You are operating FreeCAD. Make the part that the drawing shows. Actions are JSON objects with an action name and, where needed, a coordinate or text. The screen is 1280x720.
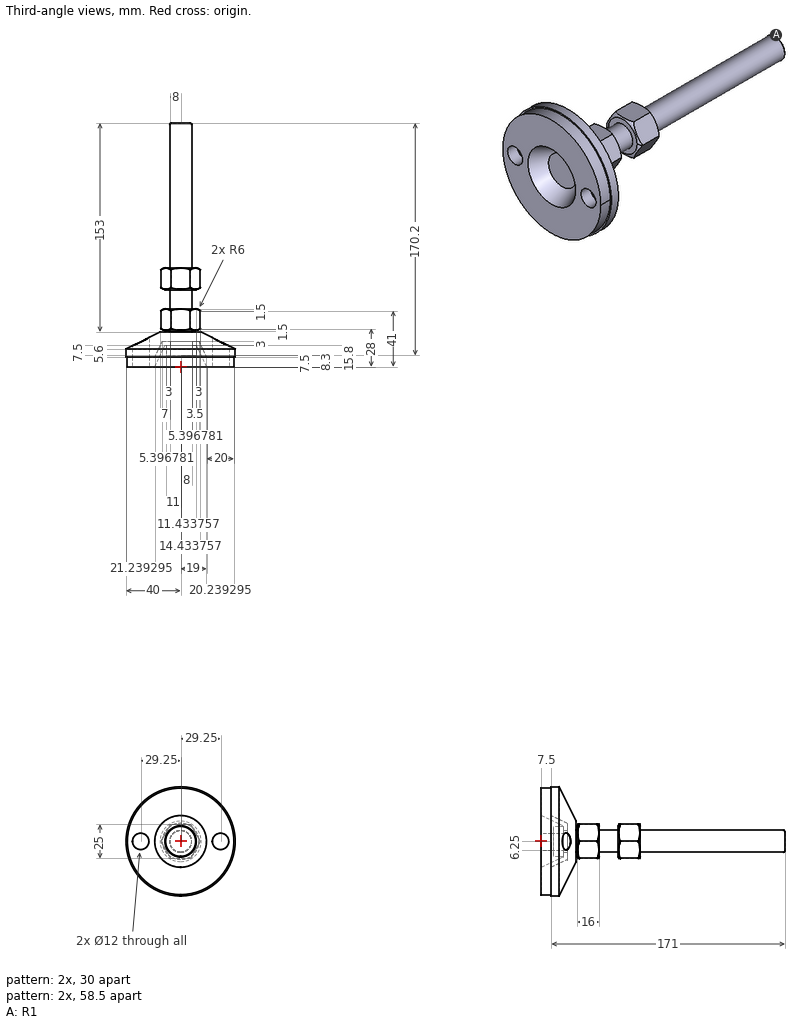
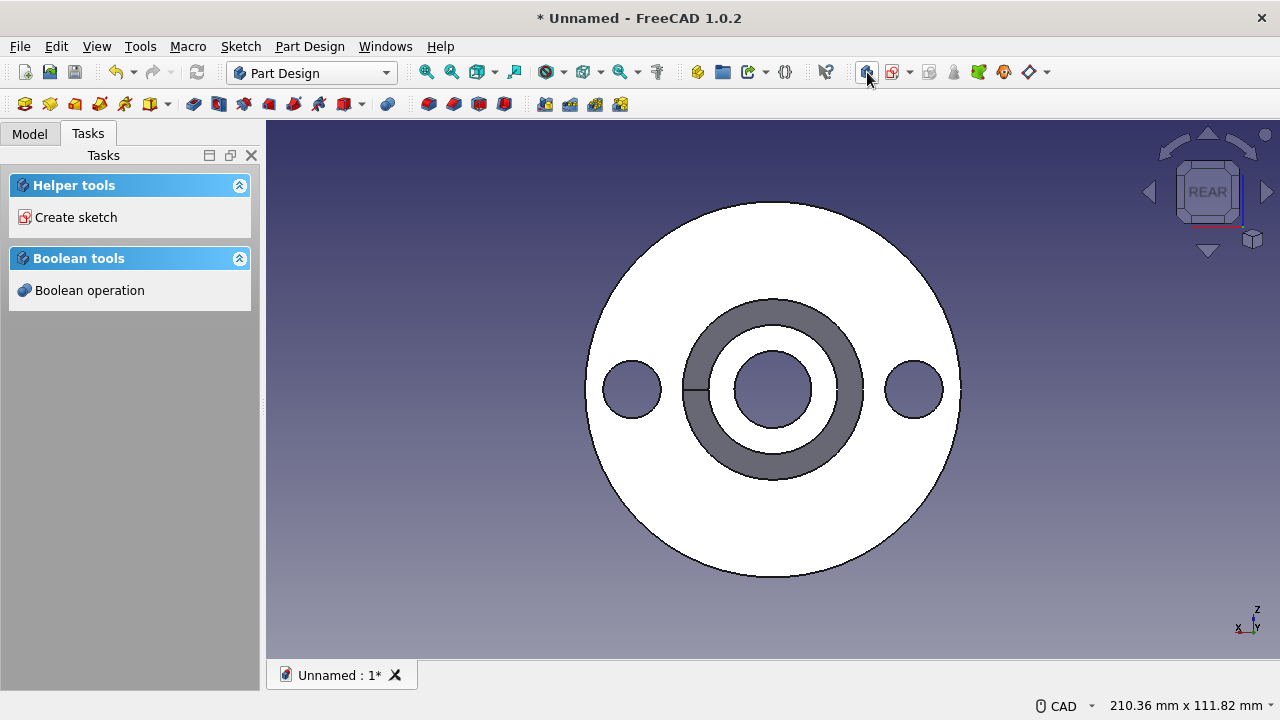
{"action": "left_click", "coordinate": [306, 619]}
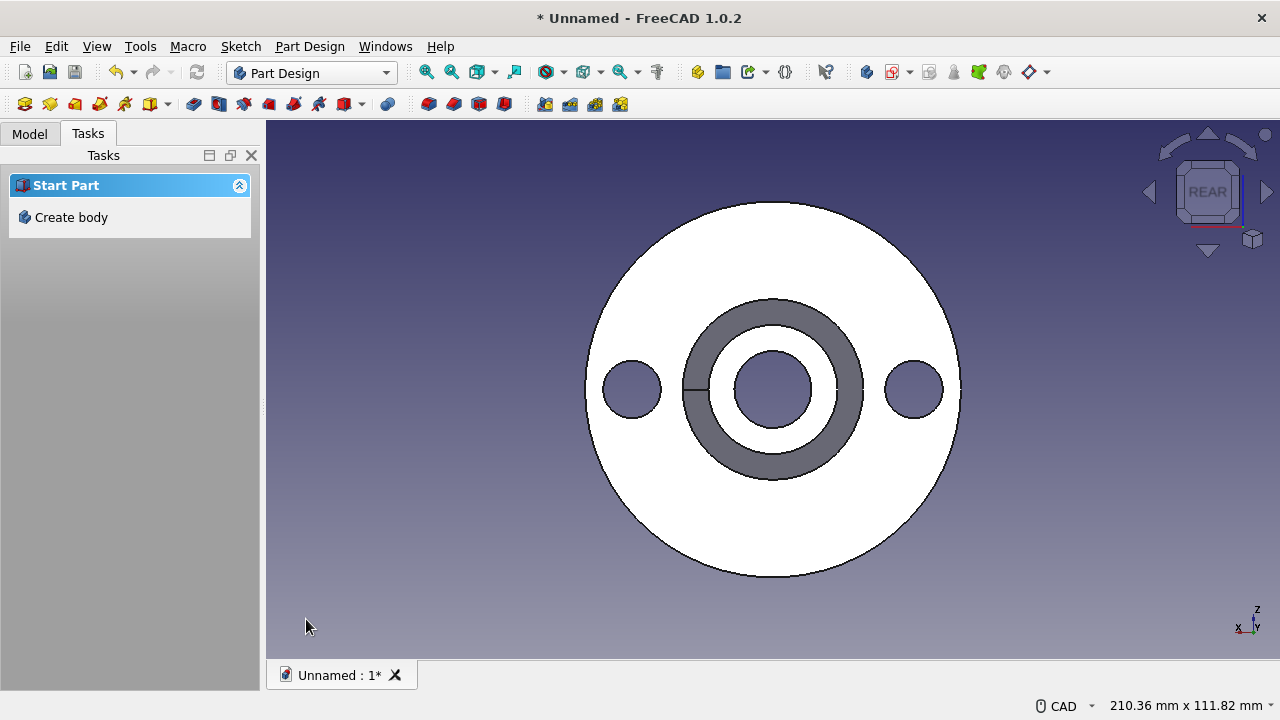
{"action": "left_click", "coordinate": [892, 72]}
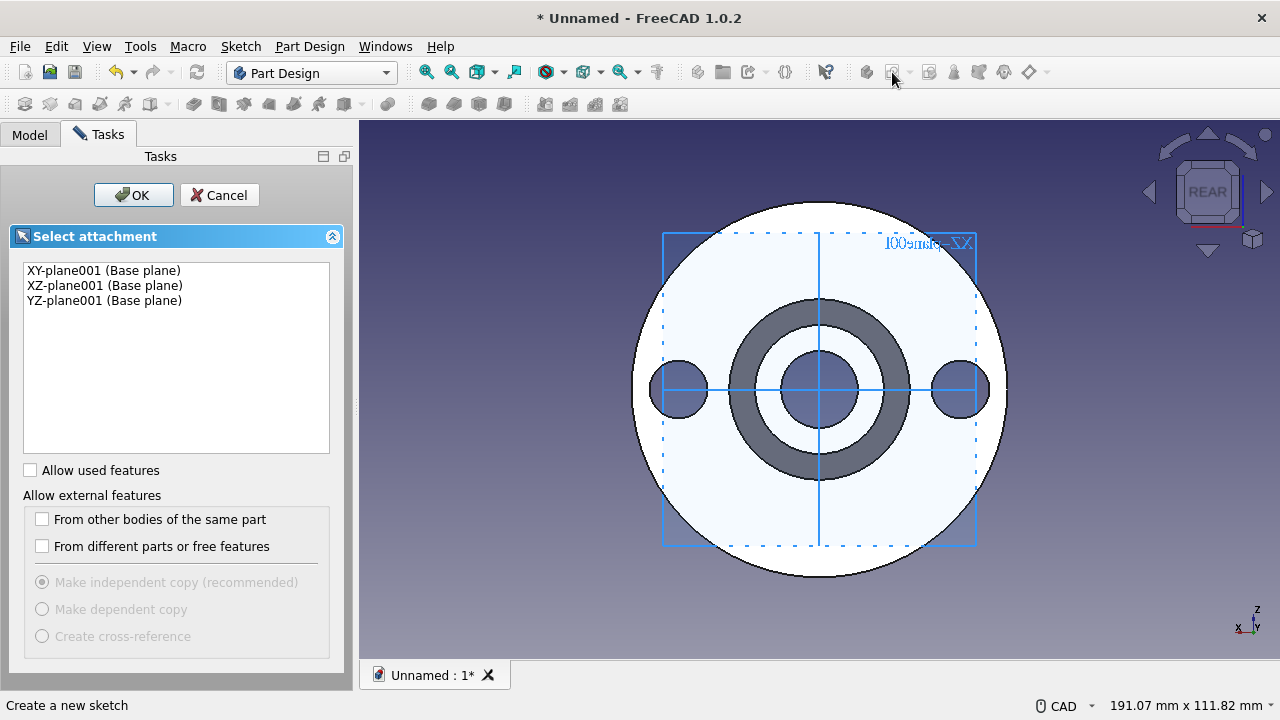
{"action": "left_click", "coordinate": [84, 270]}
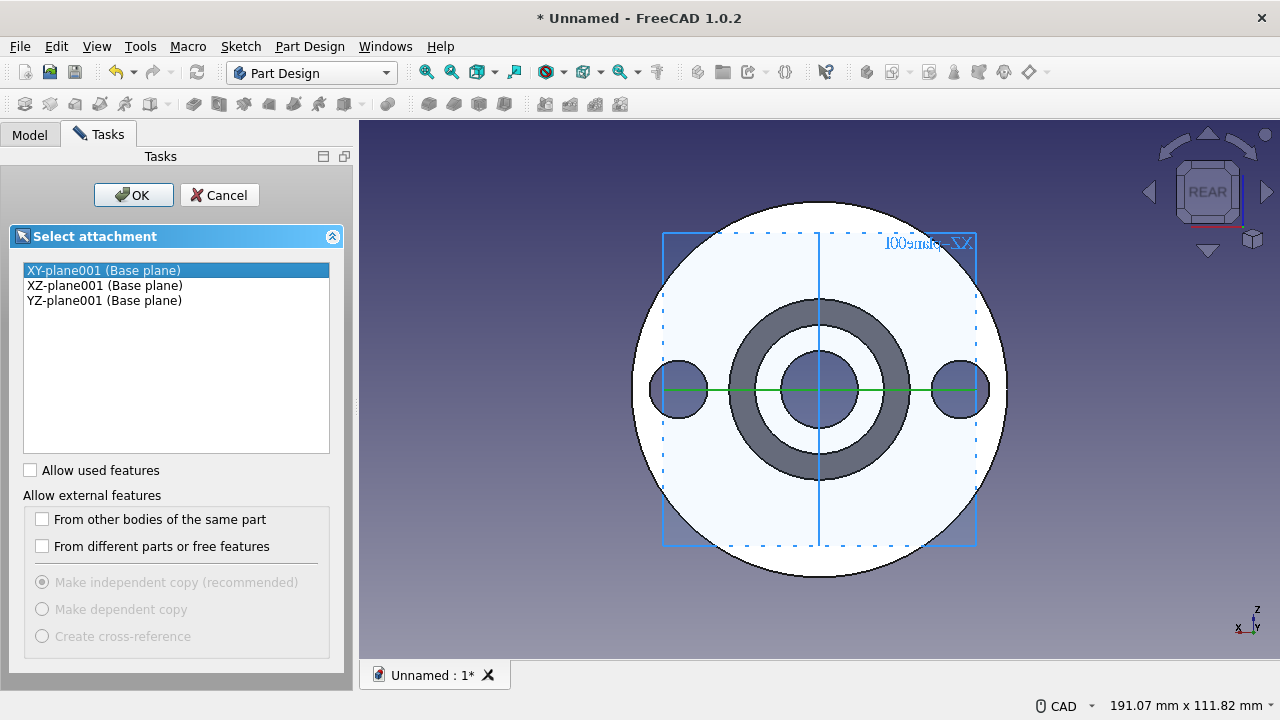
{"action": "left_click", "coordinate": [134, 195]}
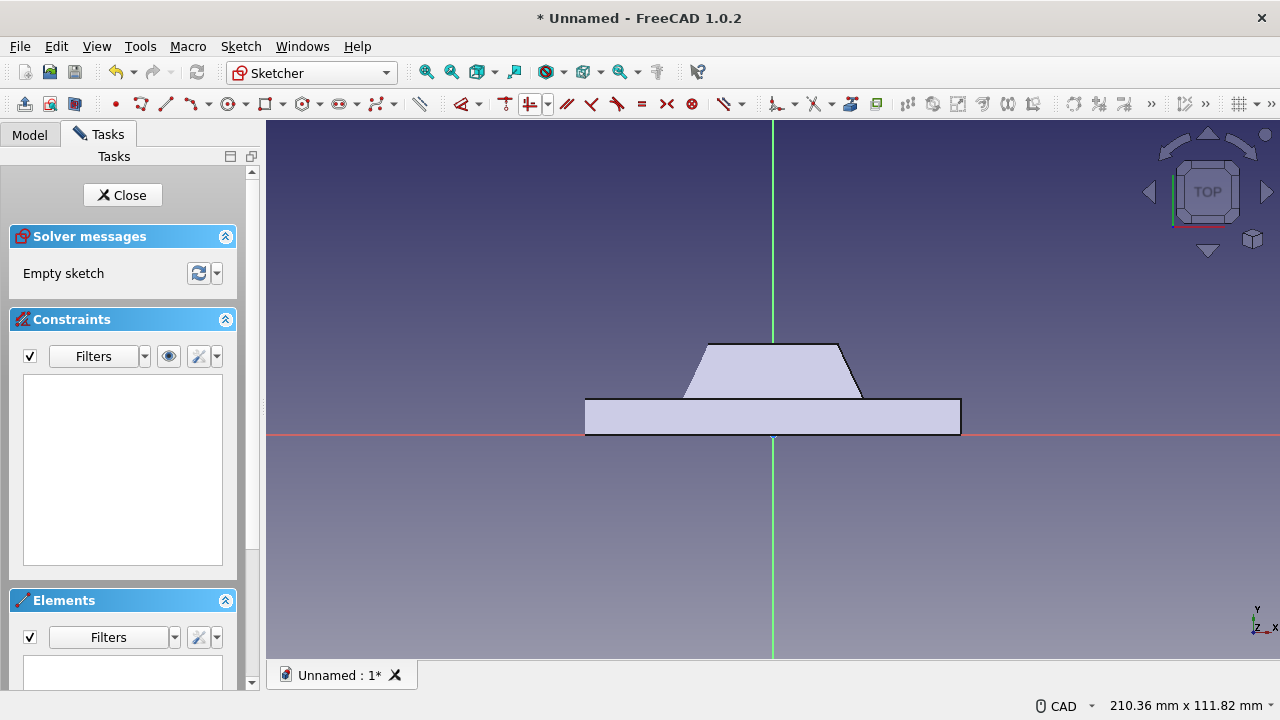
{"action": "scroll", "coordinate": [721, 614], "scroll_direction": "down", "scroll_amount": 5}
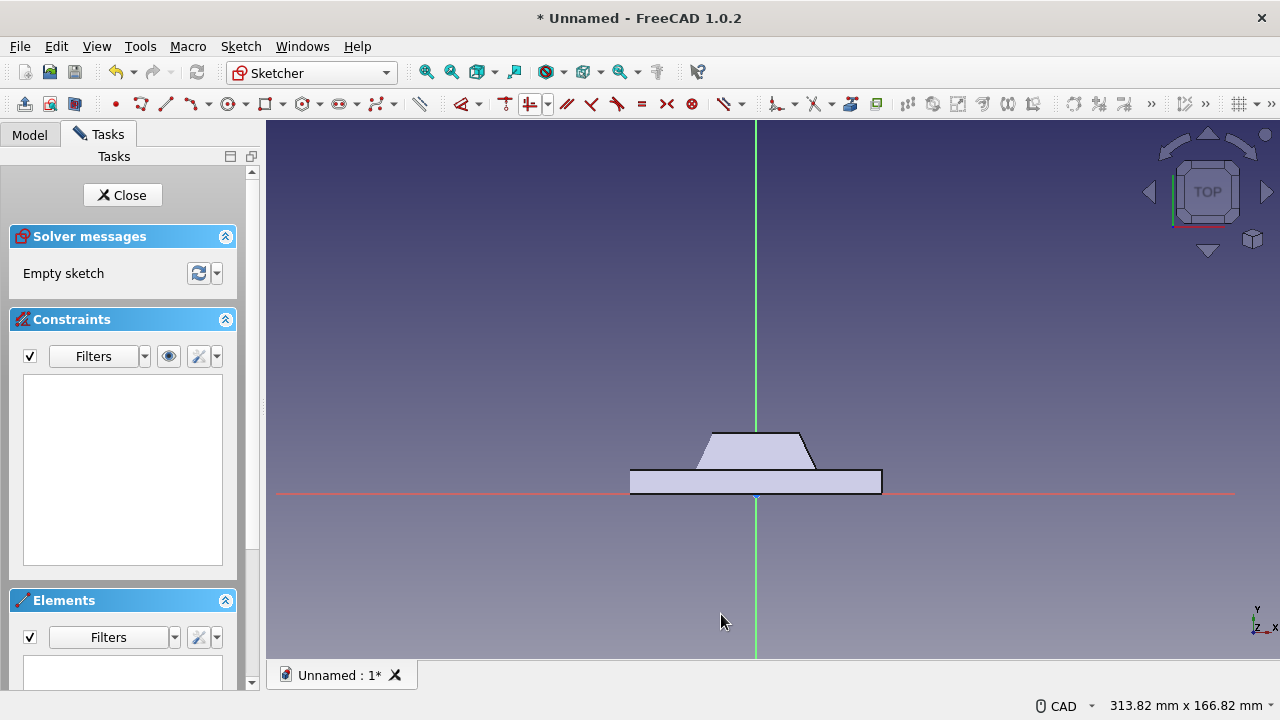
{"action": "left_click", "coordinate": [141, 104]}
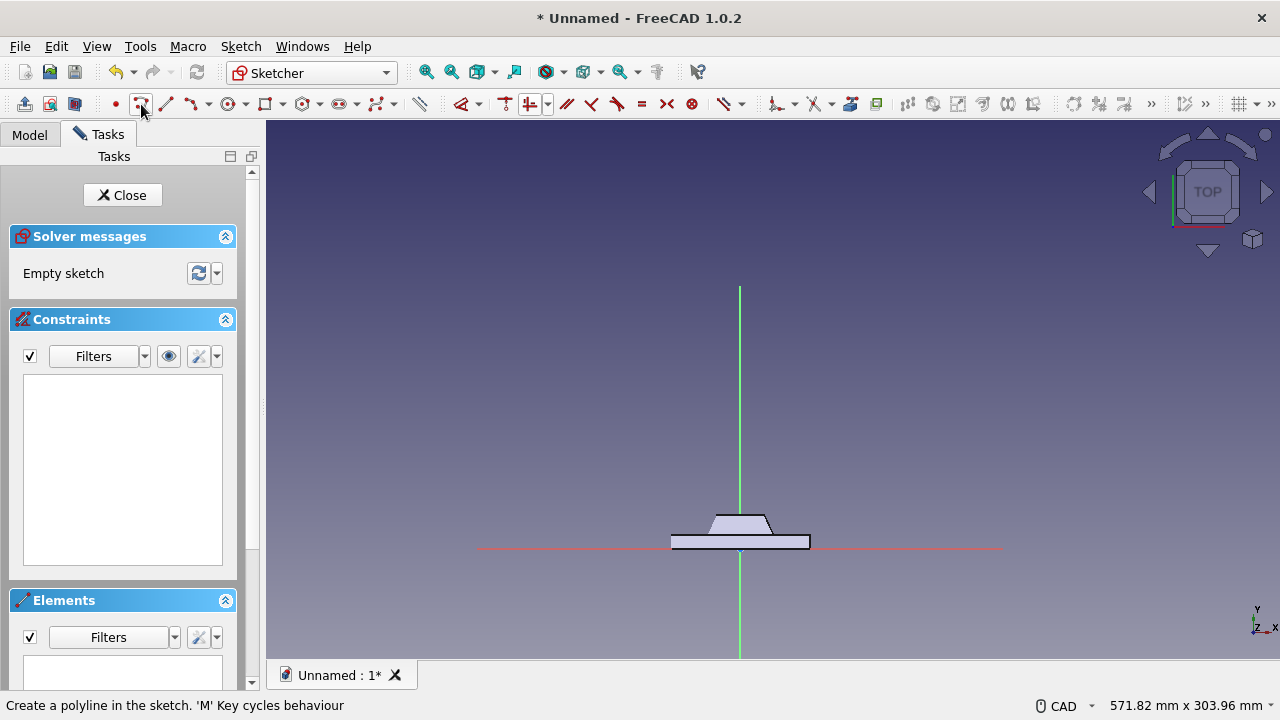
{"action": "left_click", "coordinate": [740, 534]}
{"action": "left_click", "coordinate": [731, 232]}
{"action": "left_click", "coordinate": [726, 232]}
{"action": "left_click", "coordinate": [726, 503]}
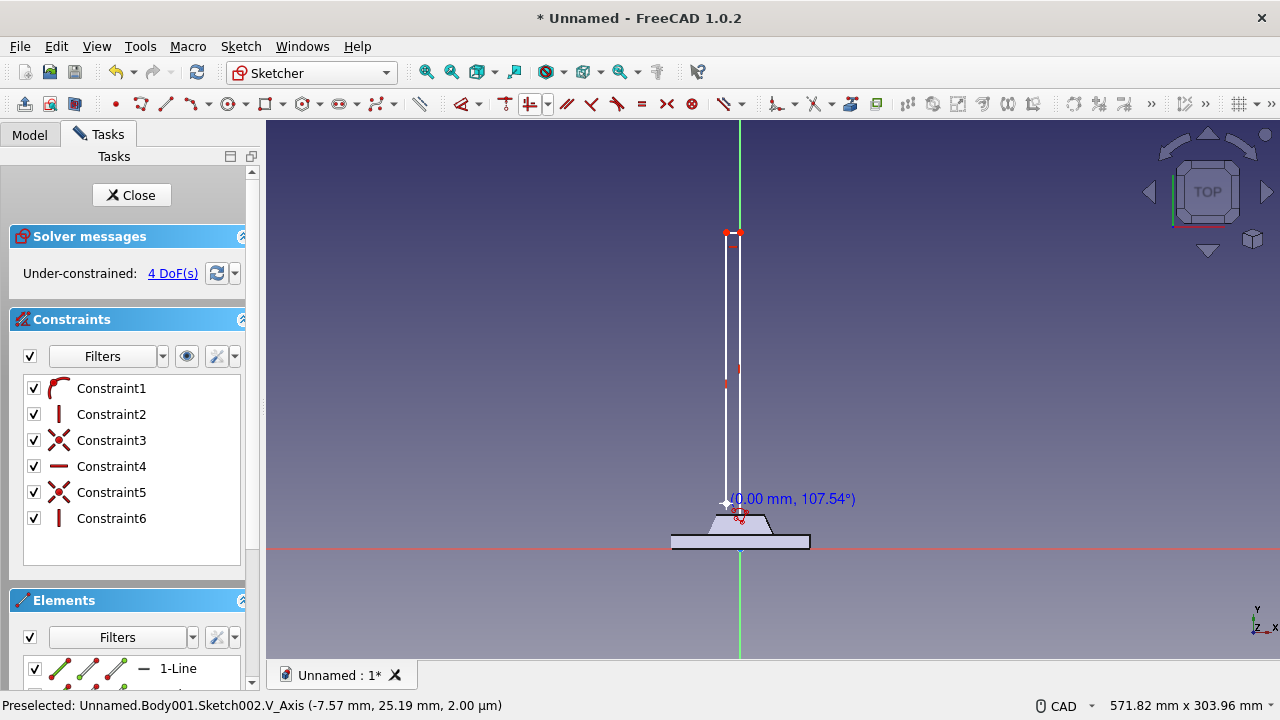
{"action": "scroll", "coordinate": [714, 503], "scroll_direction": "up", "scroll_amount": 2}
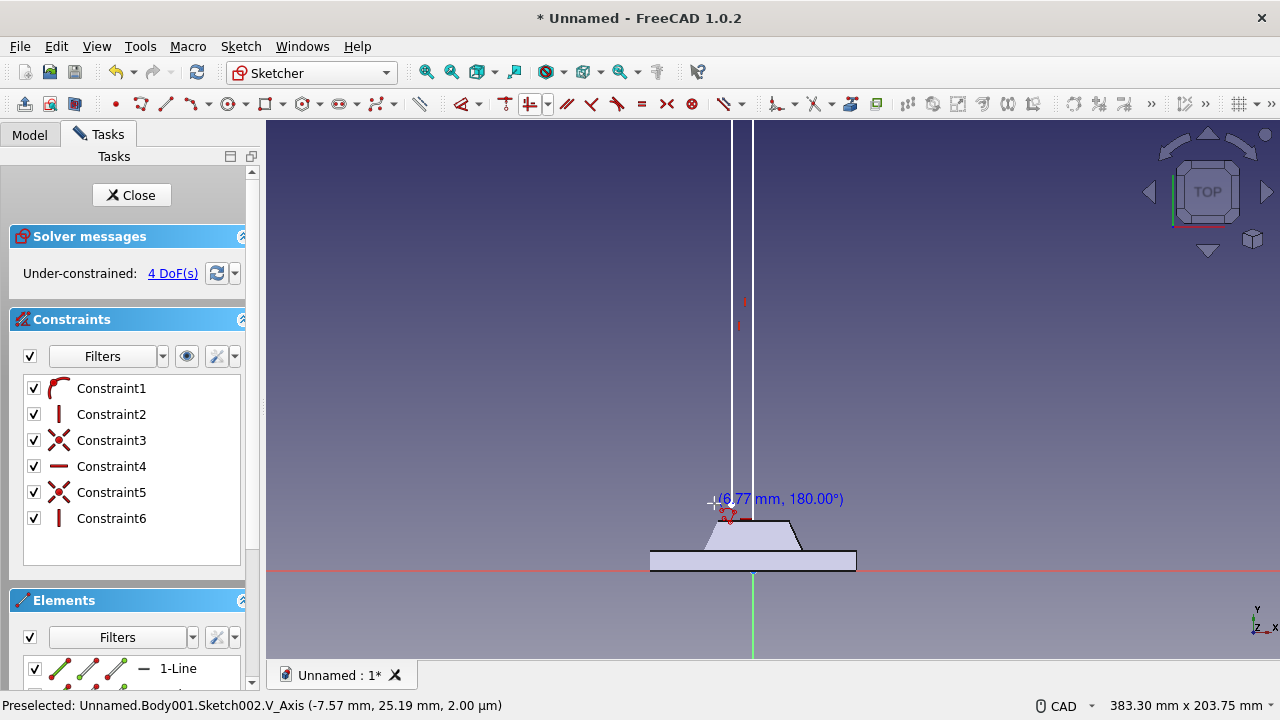
{"action": "left_click", "coordinate": [714, 503]}
{"action": "left_click", "coordinate": [647, 536]}
{"action": "left_click", "coordinate": [647, 551]}
{"action": "left_click", "coordinate": [704, 551]}
{"action": "left_click", "coordinate": [718, 521]}
{"action": "left_click", "coordinate": [732, 521]}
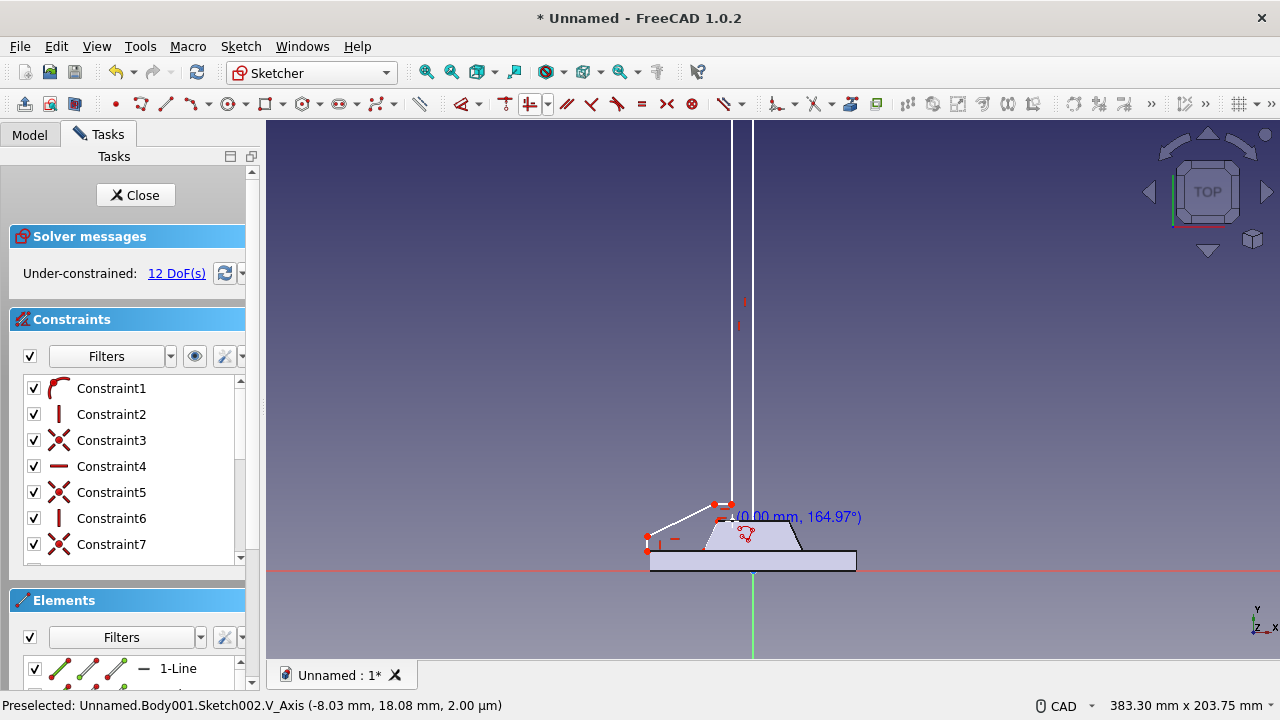
{"action": "scroll", "coordinate": [732, 529], "scroll_direction": "up", "scroll_amount": 4}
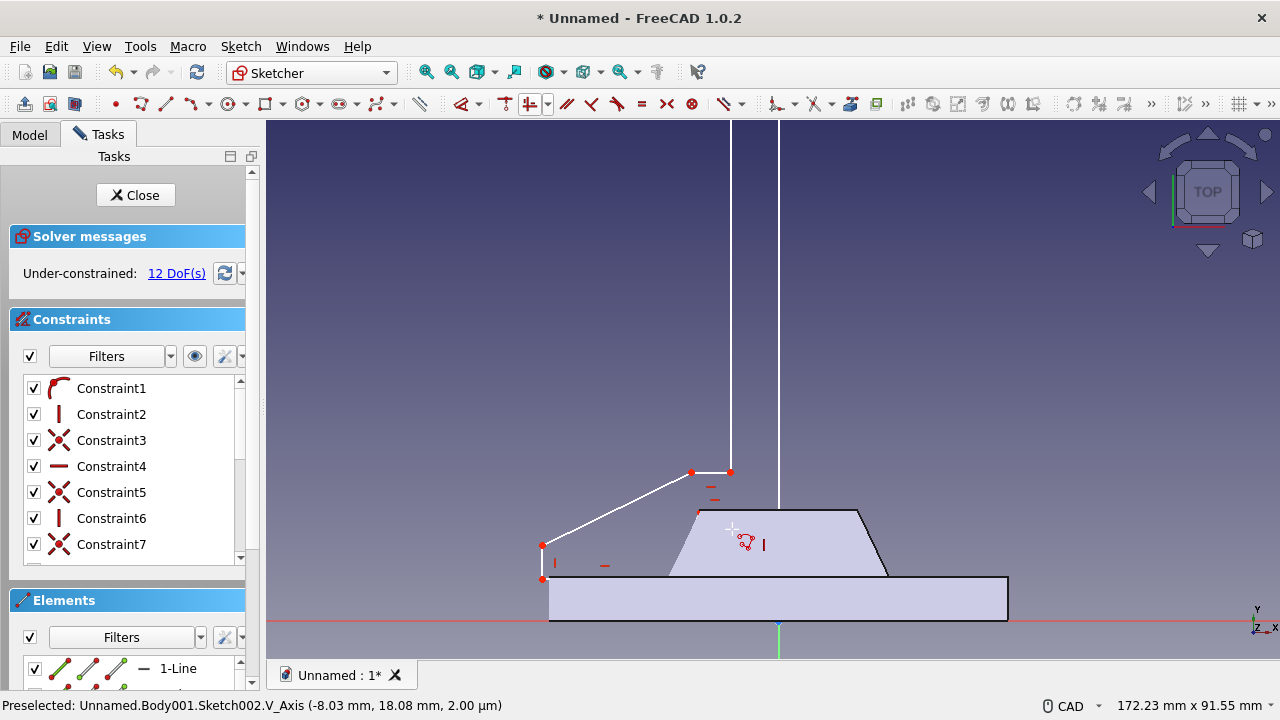
{"action": "left_click", "coordinate": [731, 528]}
{"action": "left_click", "coordinate": [714, 528]}
{"action": "left_click", "coordinate": [714, 572]}
{"action": "left_click", "coordinate": [779, 576]}
{"action": "key", "text": "Escape"}
{"action": "key", "text": "Escape"}